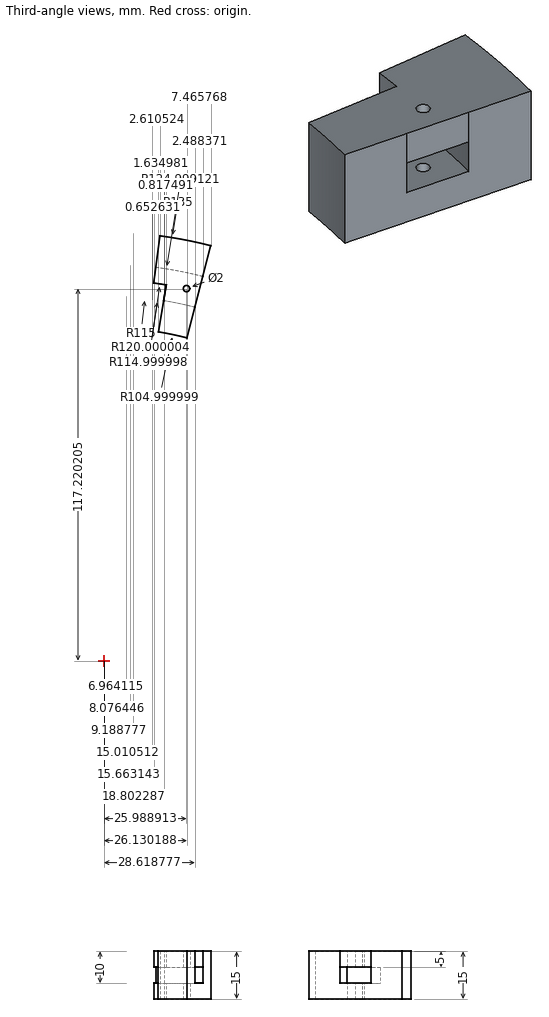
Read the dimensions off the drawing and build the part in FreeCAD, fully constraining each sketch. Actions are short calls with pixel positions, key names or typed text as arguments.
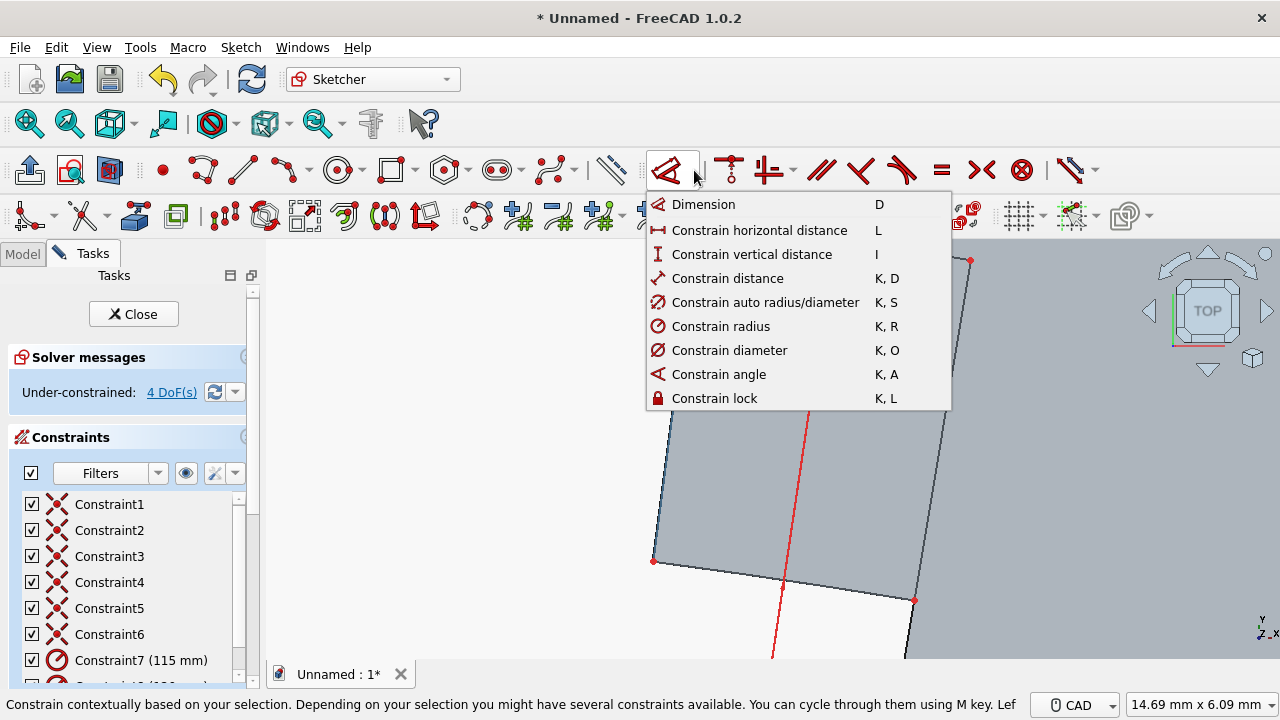
click(799, 230)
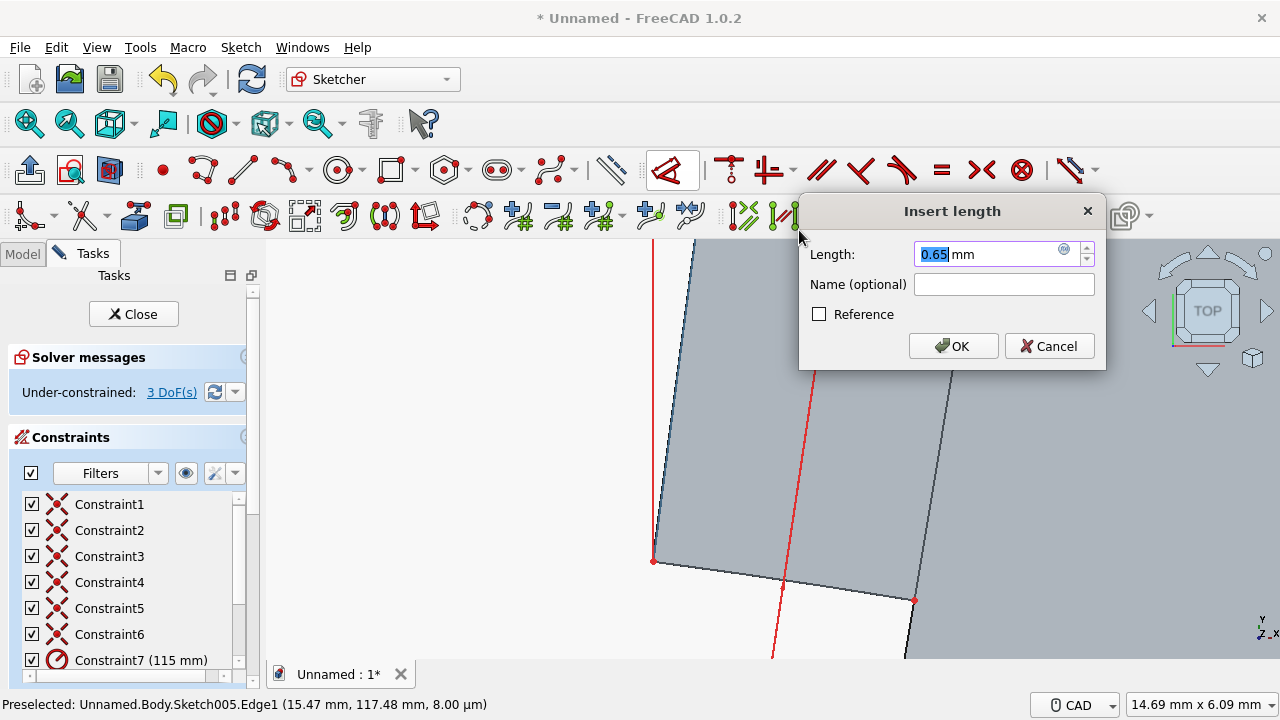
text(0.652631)
key(Return)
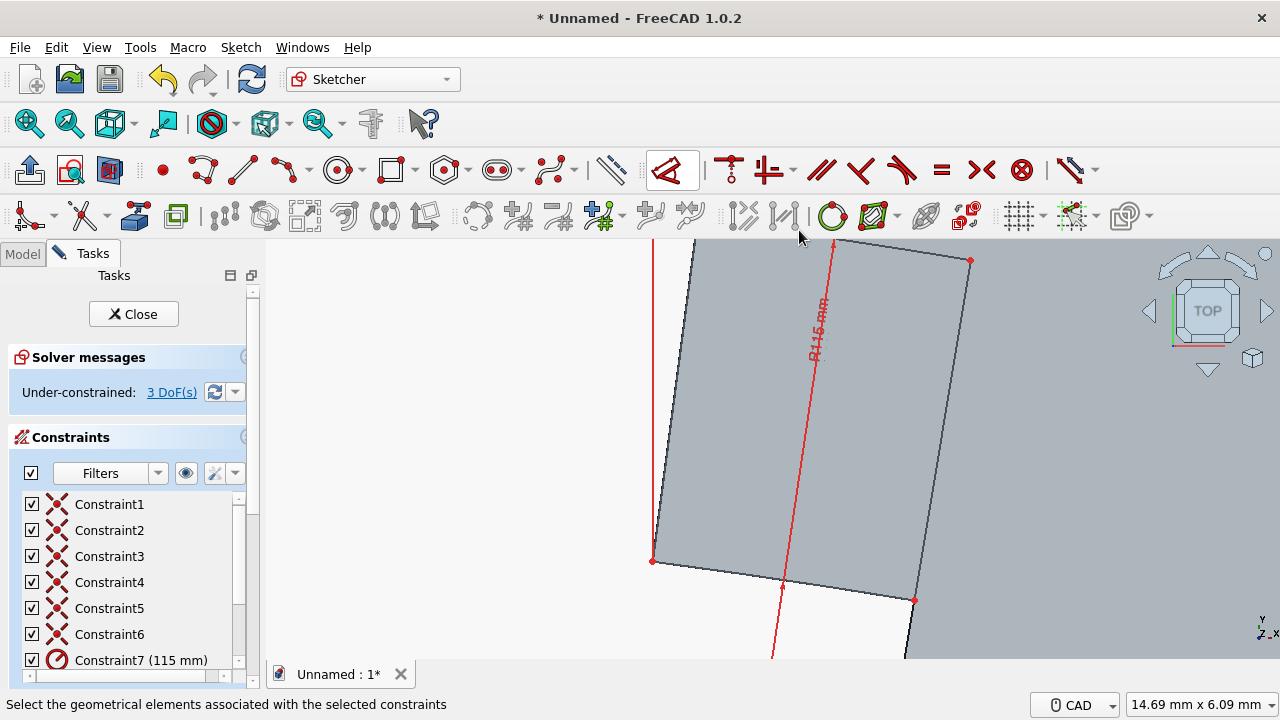
click(931, 498)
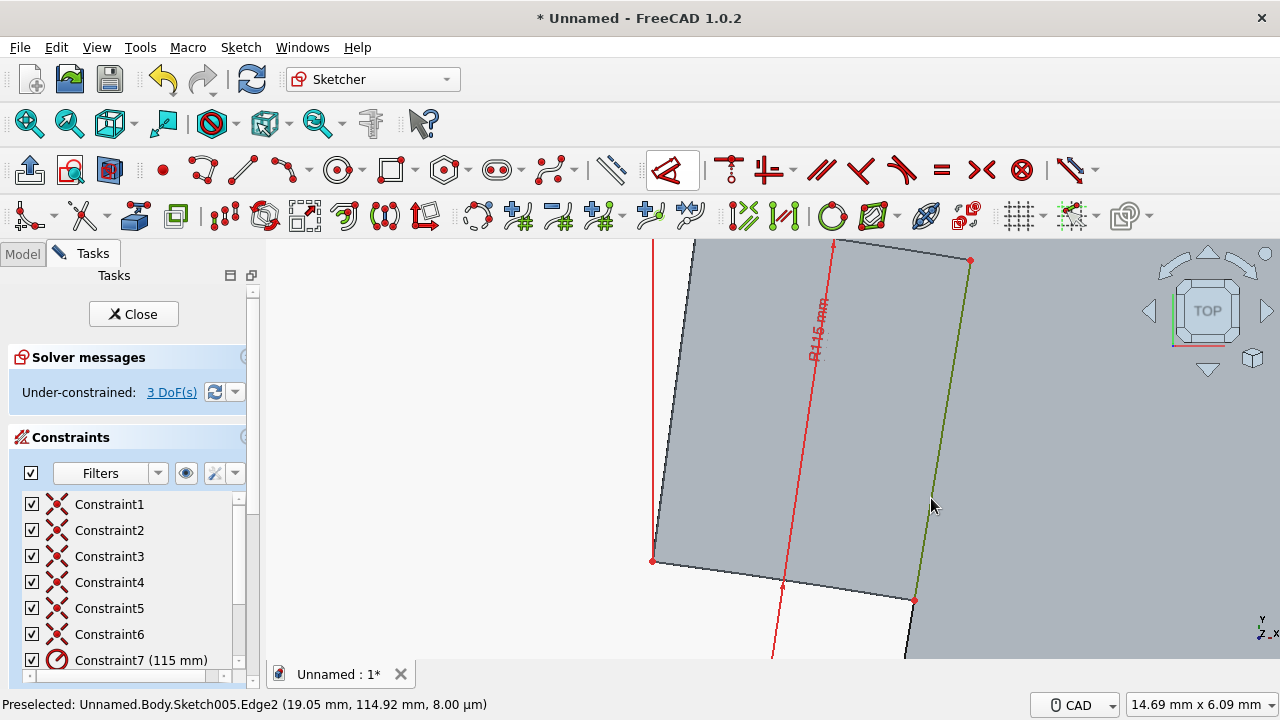
click(694, 170)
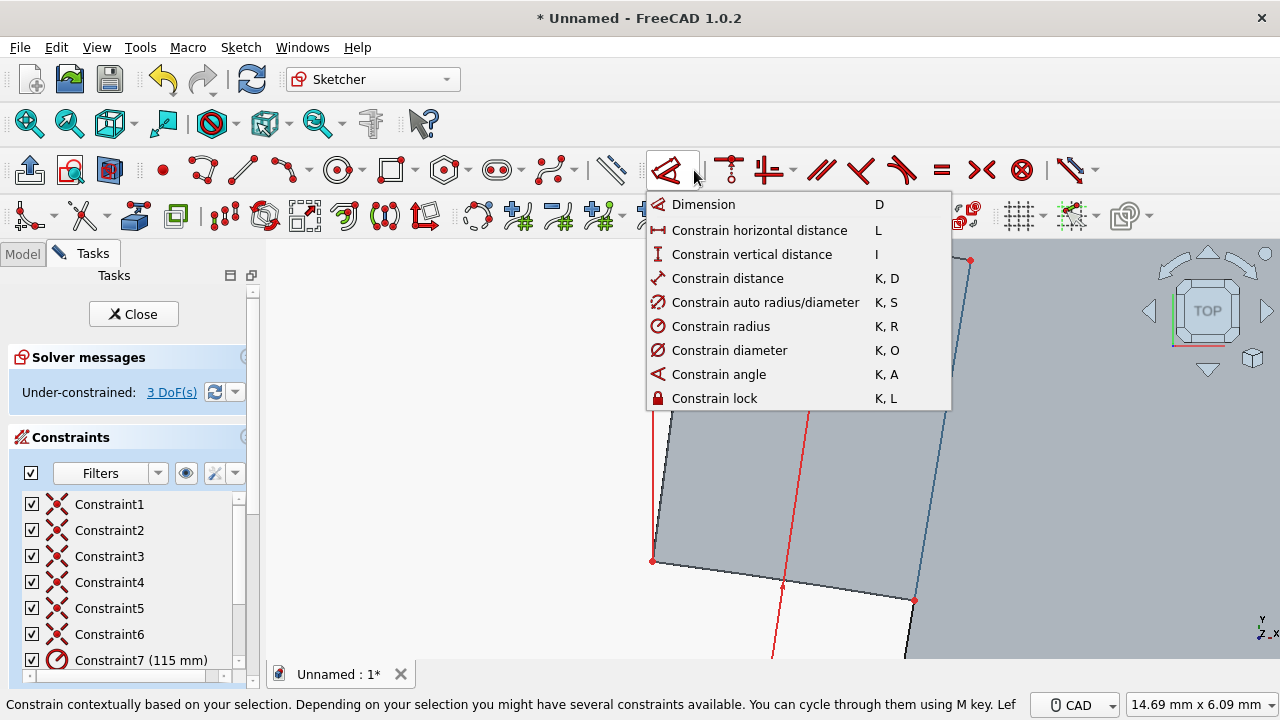
click(799, 230)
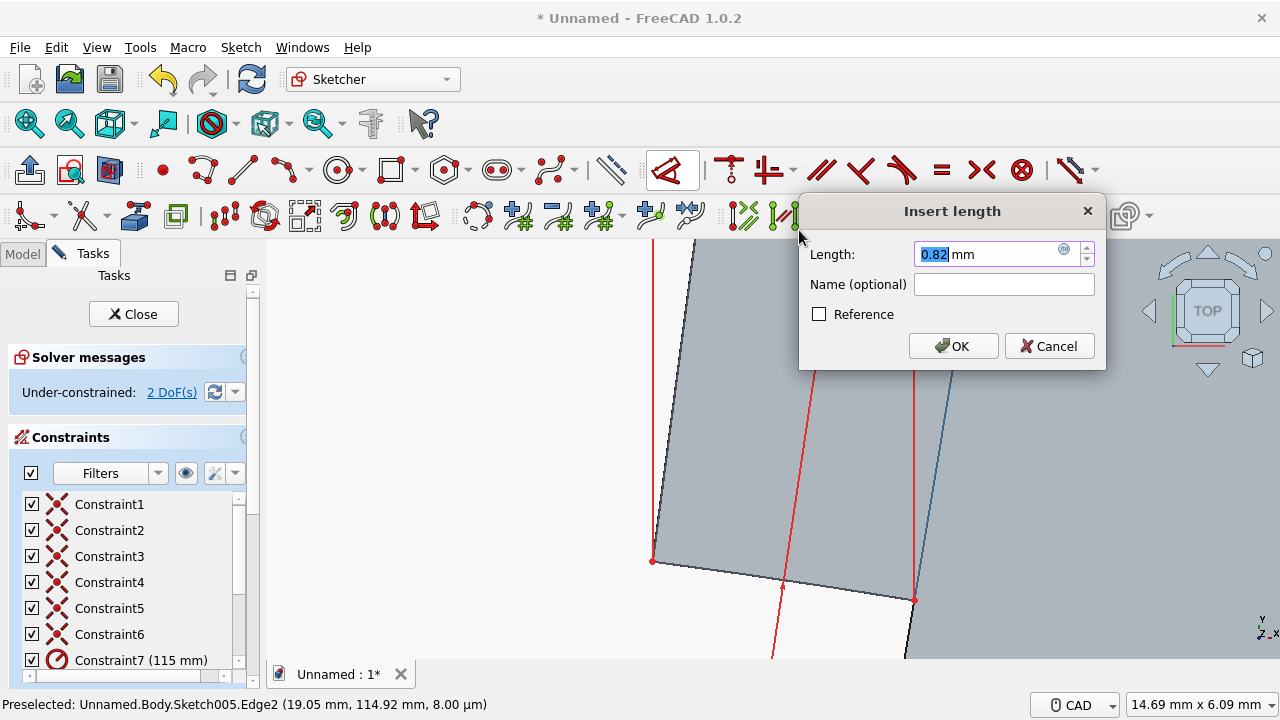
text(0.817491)
key(Return)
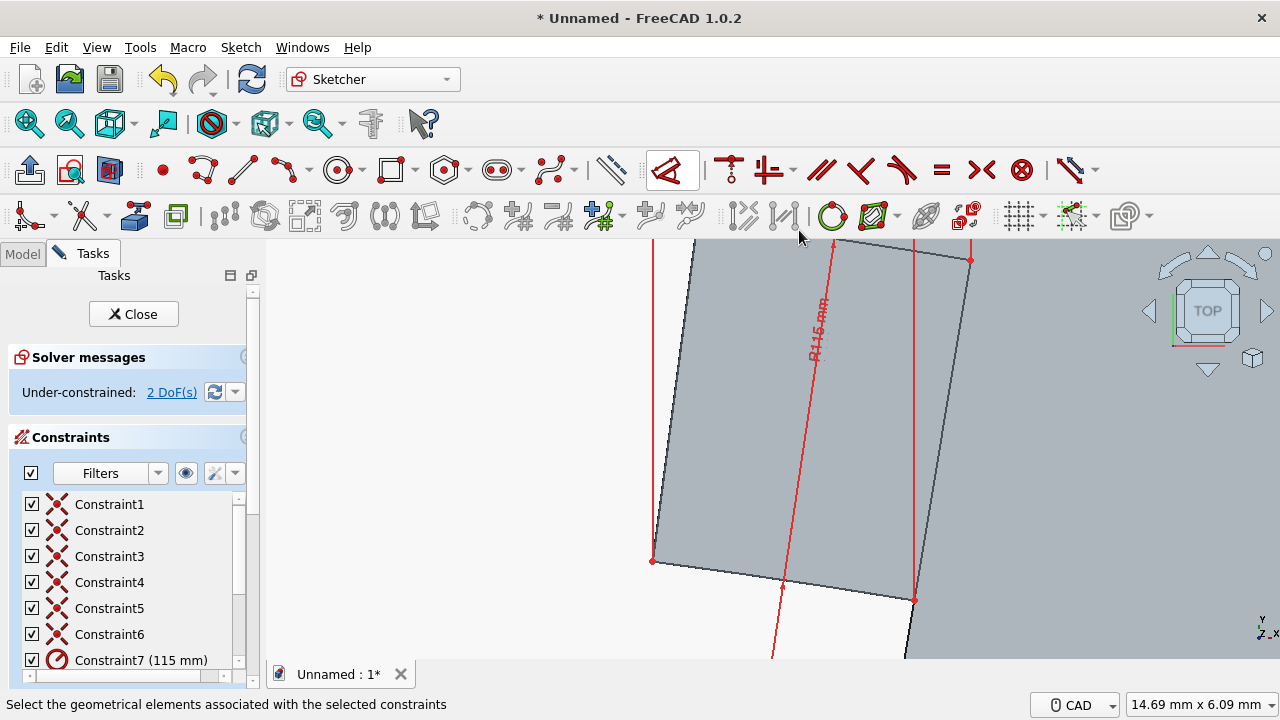
scroll(487, 528, down, 2)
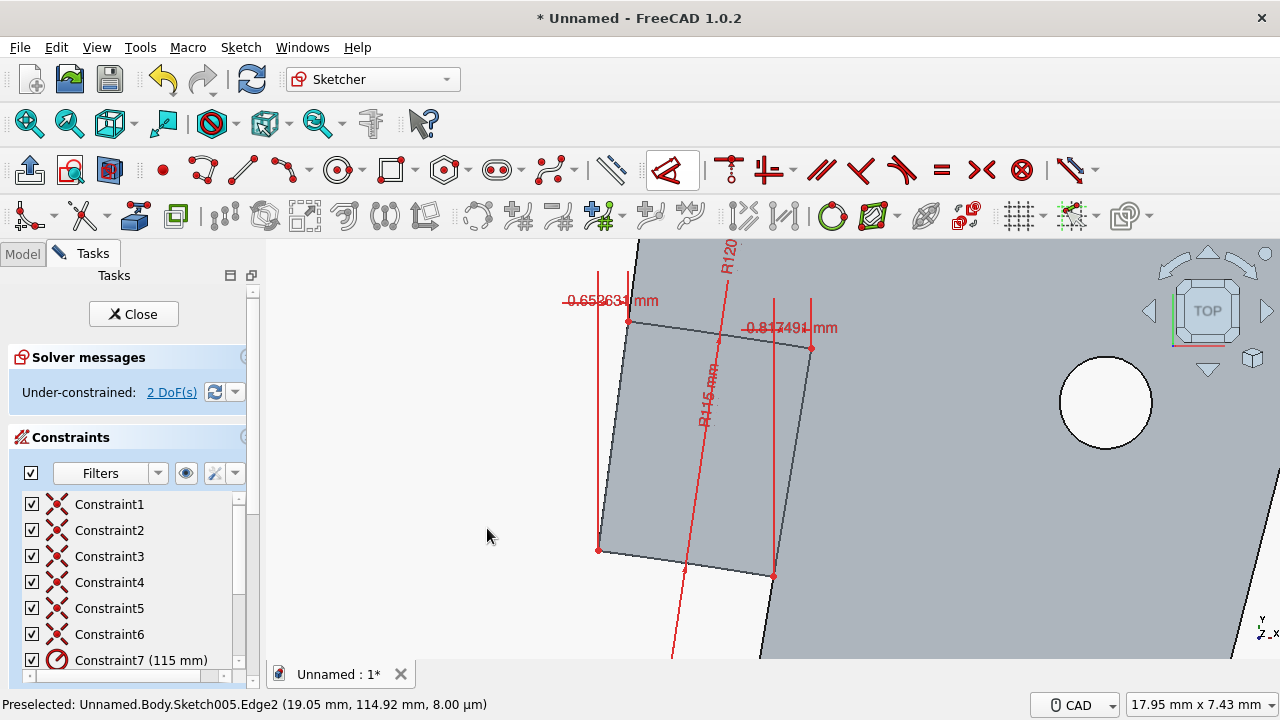
scroll(628, 322, up, 14)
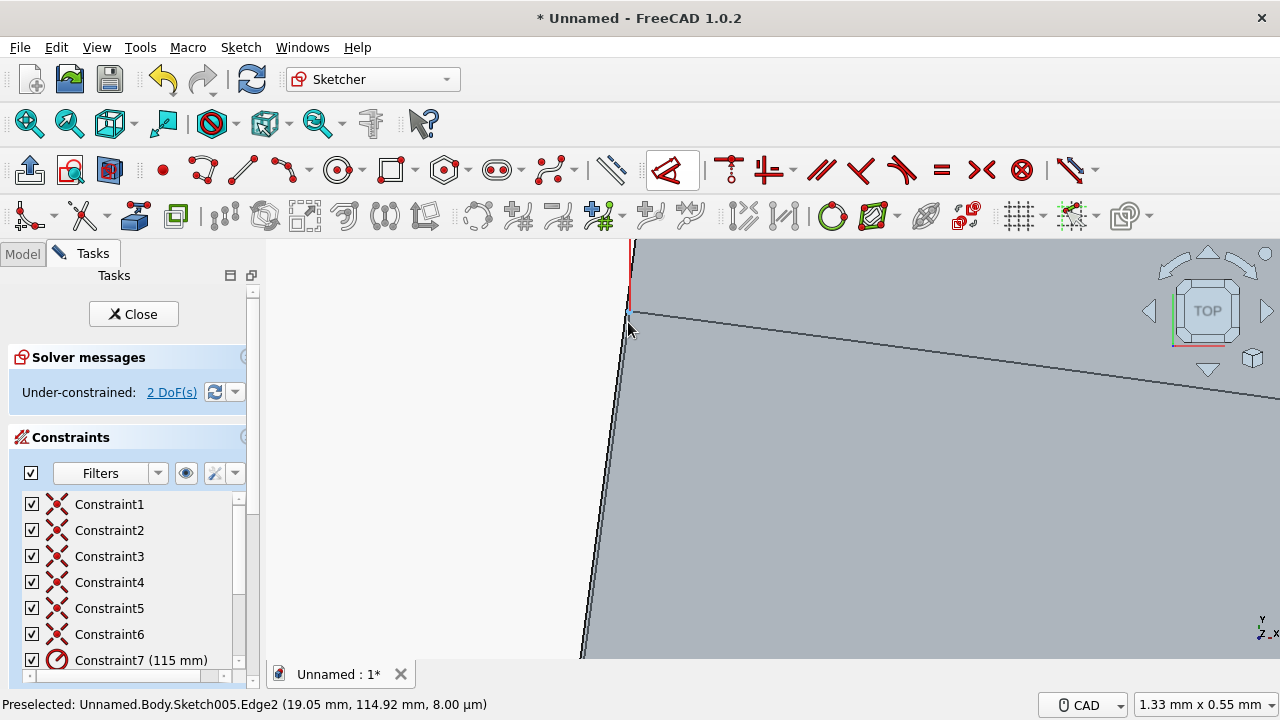
click(630, 311)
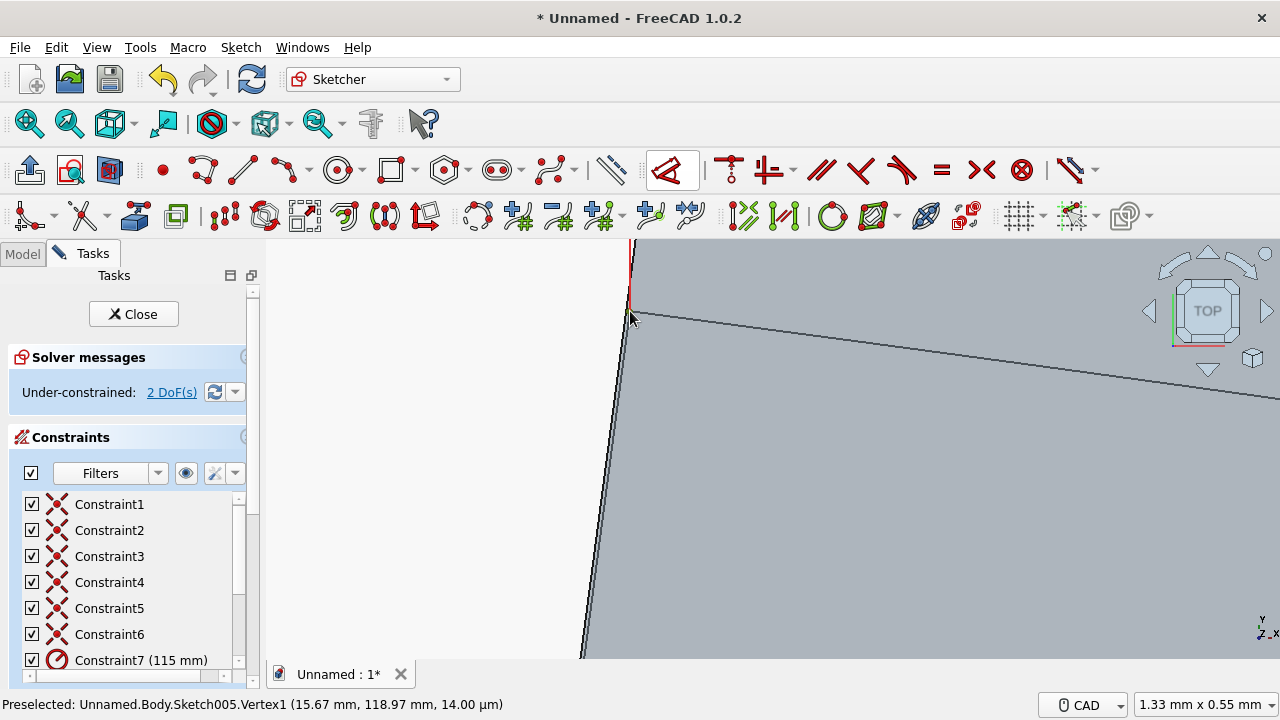
key(l)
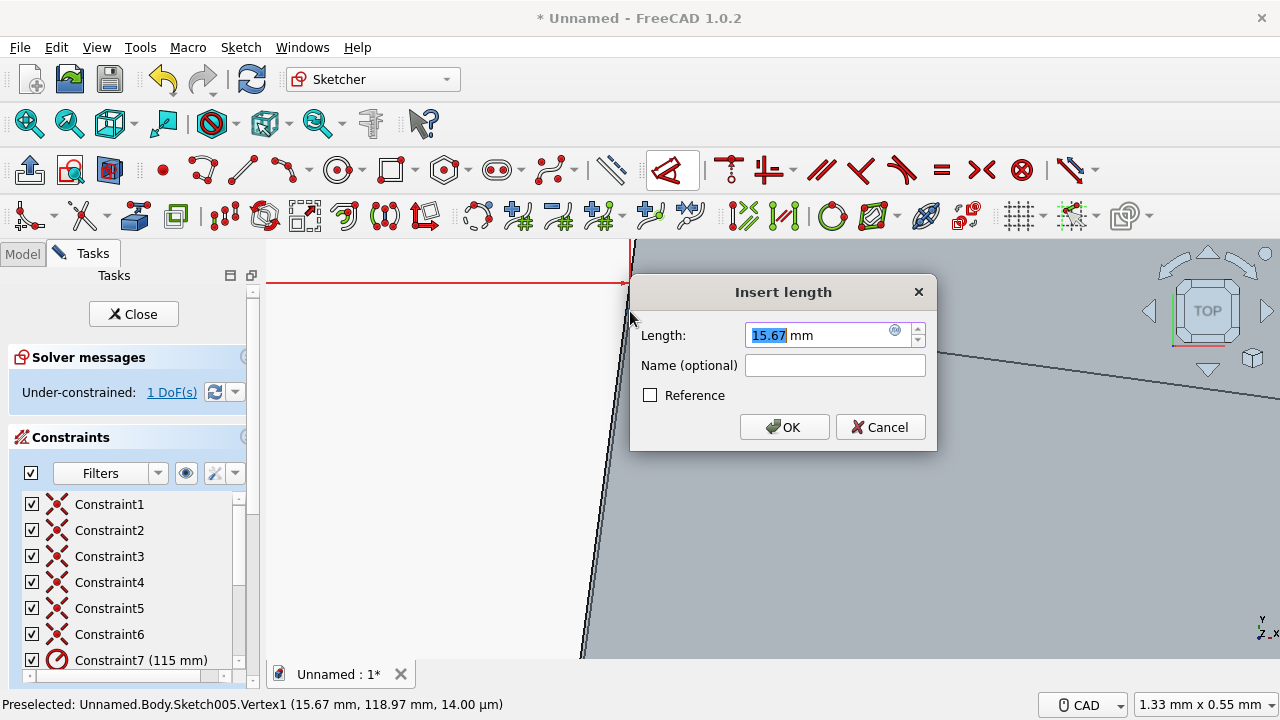
text(15.663143)
key(Return)